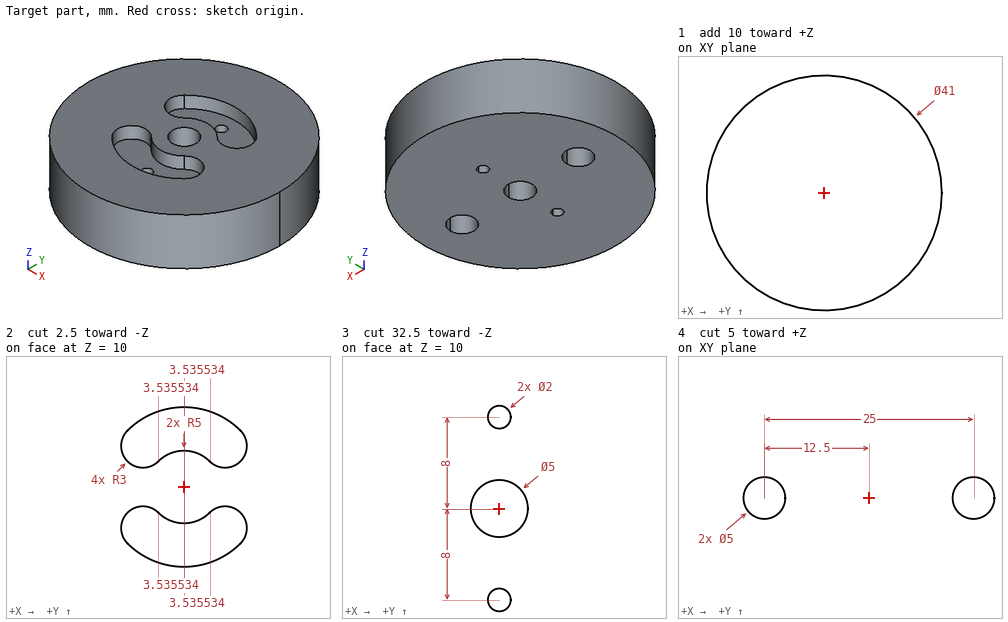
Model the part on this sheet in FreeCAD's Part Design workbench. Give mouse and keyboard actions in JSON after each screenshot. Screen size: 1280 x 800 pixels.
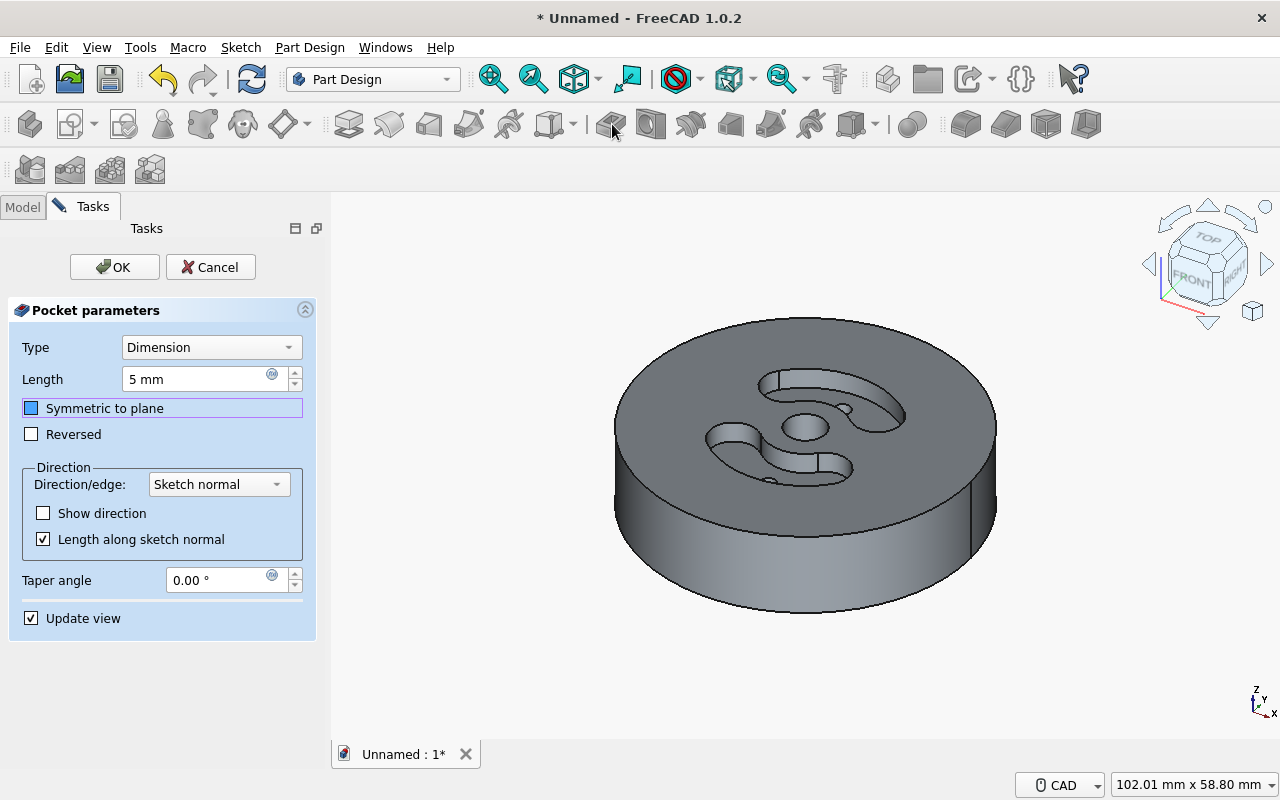
{"action": "left_click", "coordinate": [30, 434]}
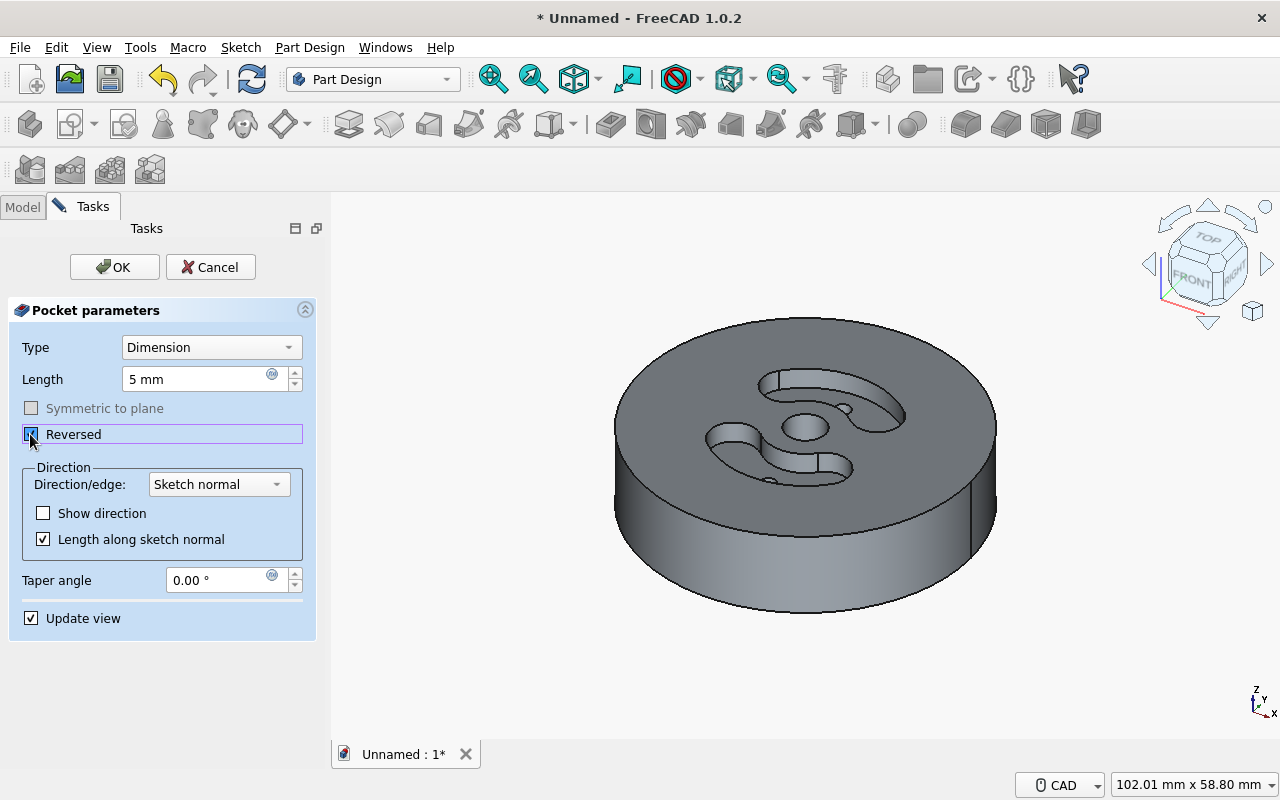
{"action": "left_click", "coordinate": [115, 267]}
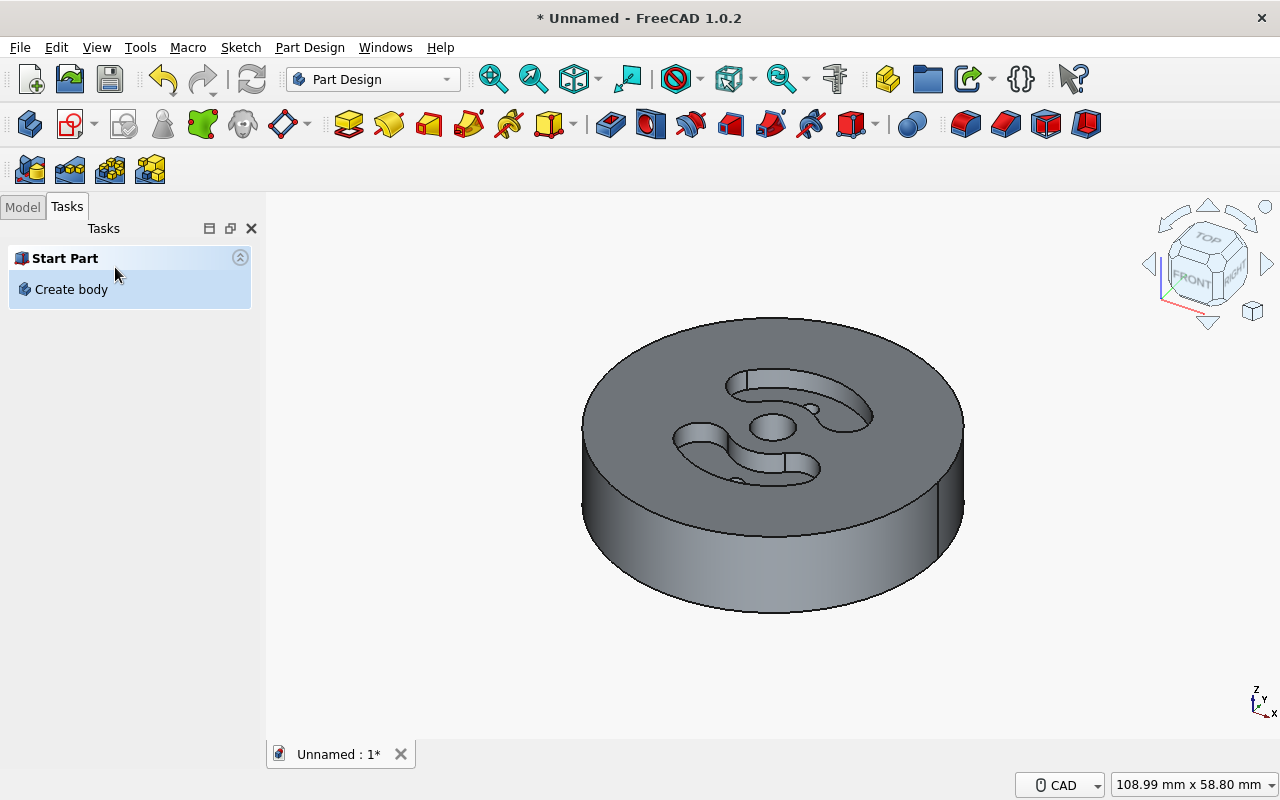
{"action": "key", "text": "0"}